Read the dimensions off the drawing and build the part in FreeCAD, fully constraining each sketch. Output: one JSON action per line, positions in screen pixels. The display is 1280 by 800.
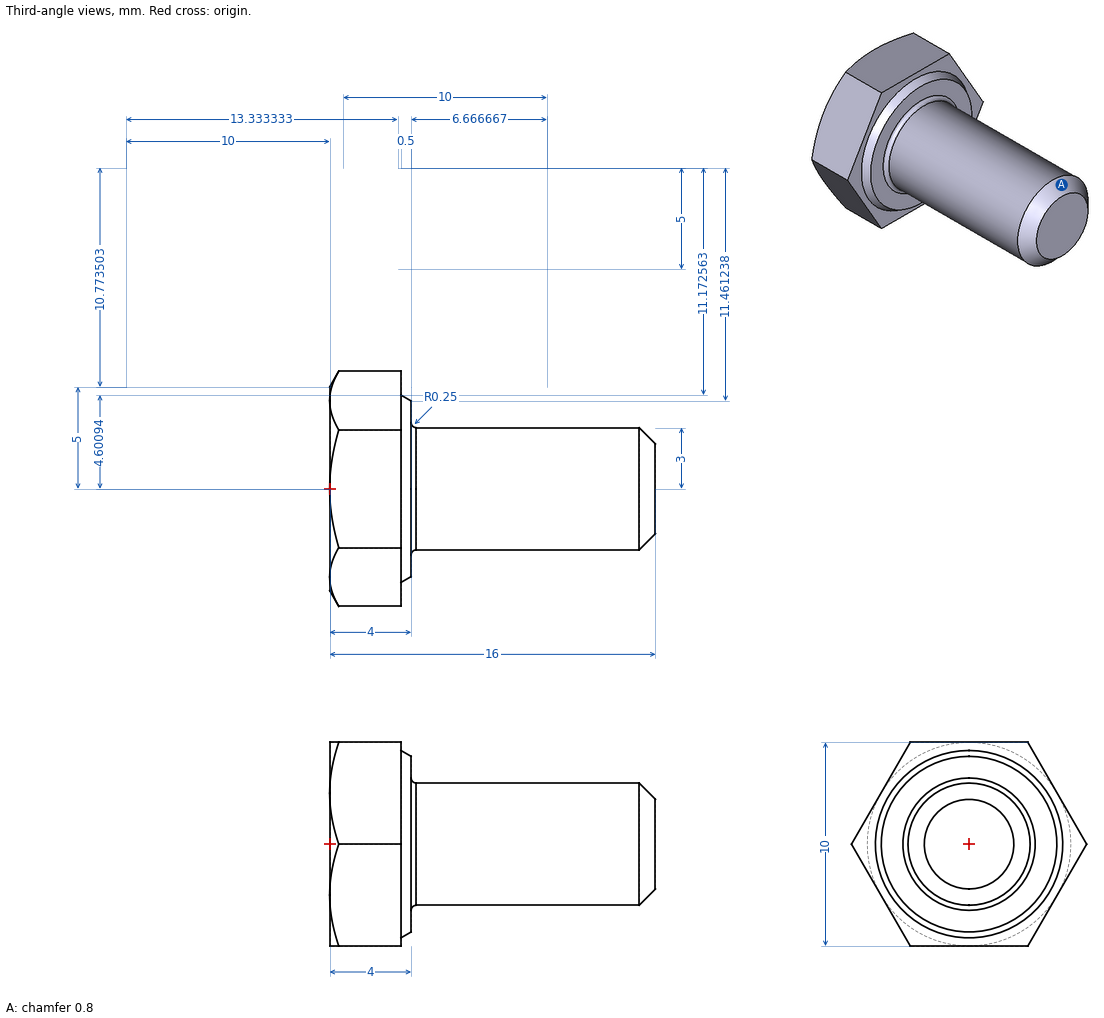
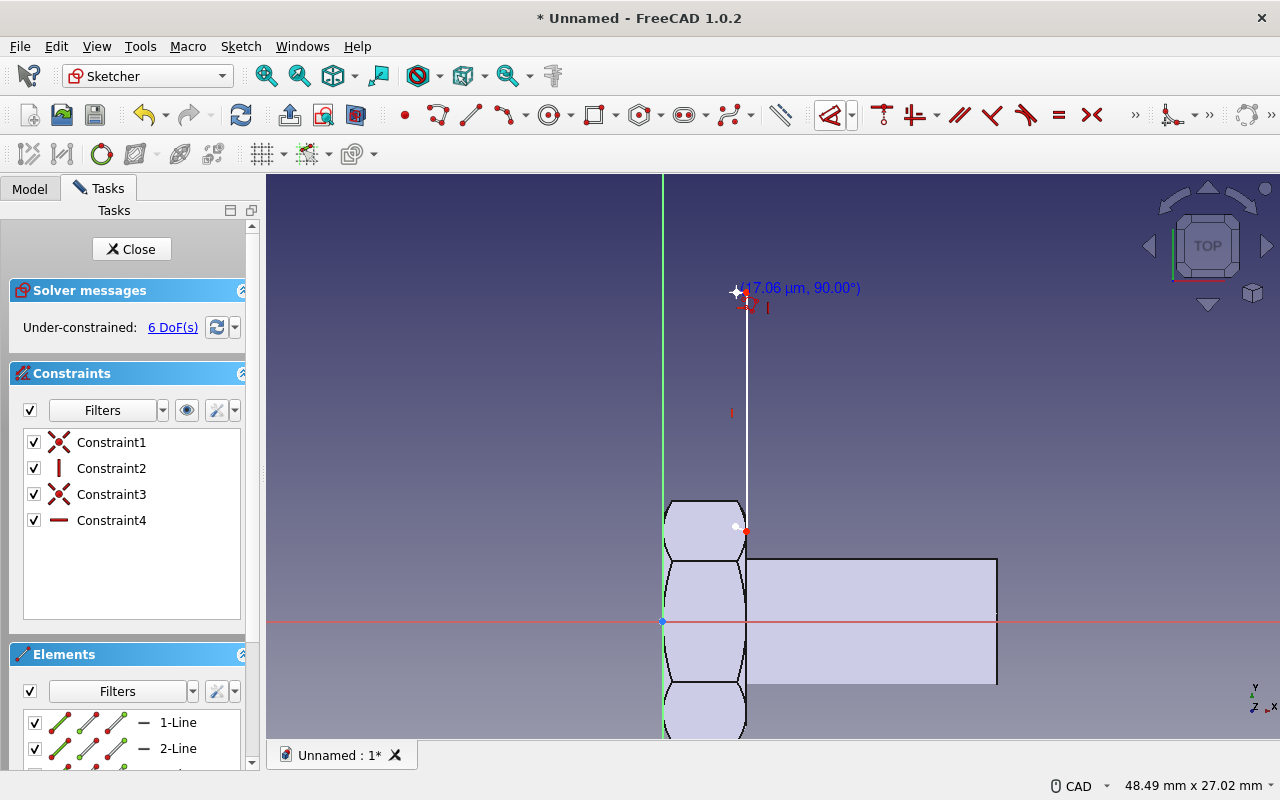
{"action": "scroll", "coordinate": [736, 525], "scroll_direction": "up", "scroll_amount": 5}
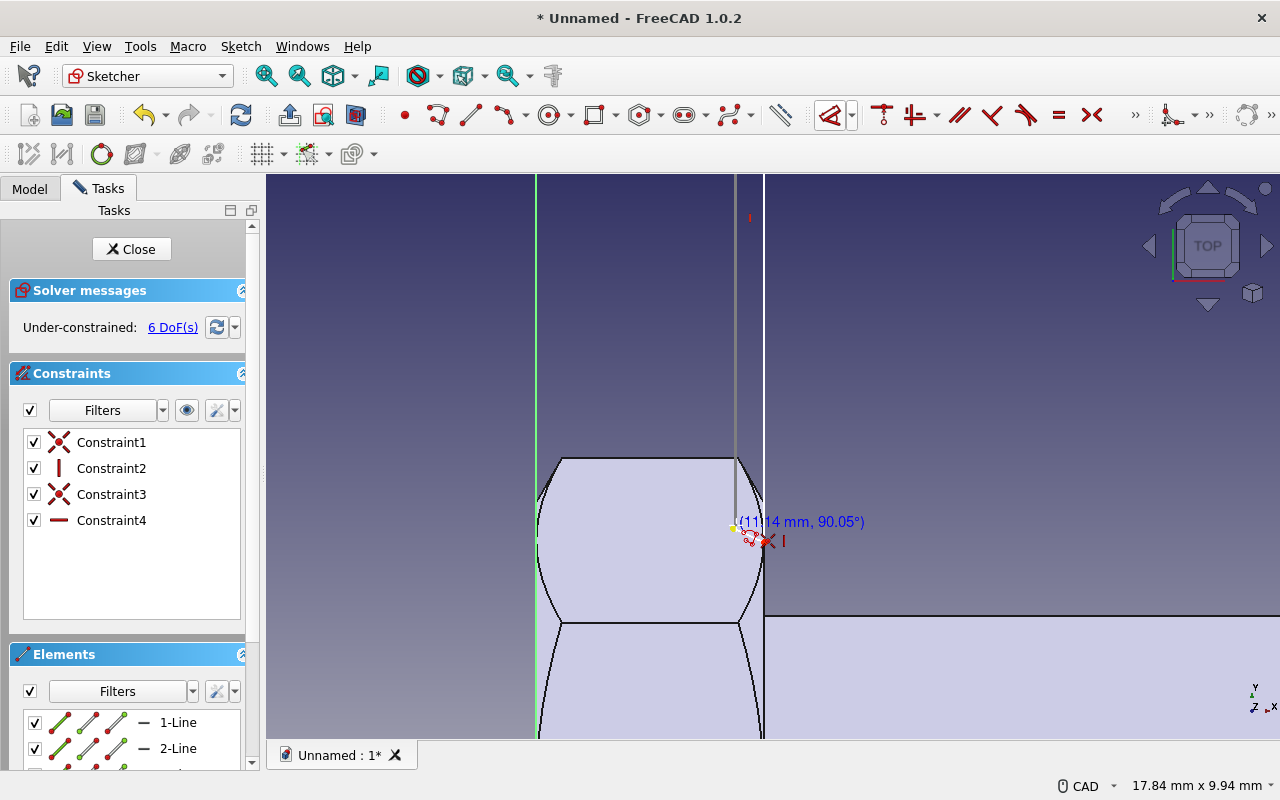
{"action": "left_click", "coordinate": [734, 529]}
{"action": "key", "text": "Escape"}
{"action": "key", "text": "Escape"}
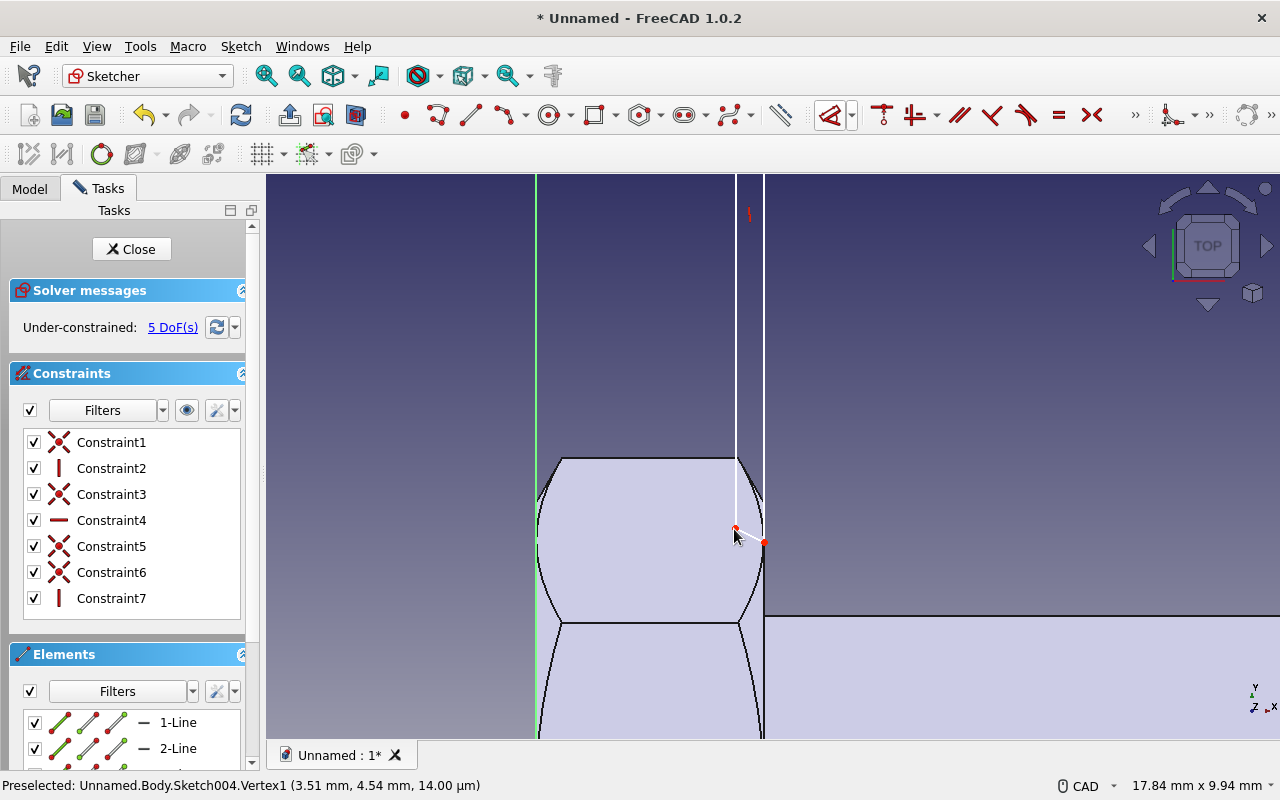
{"action": "left_click", "coordinate": [764, 543]}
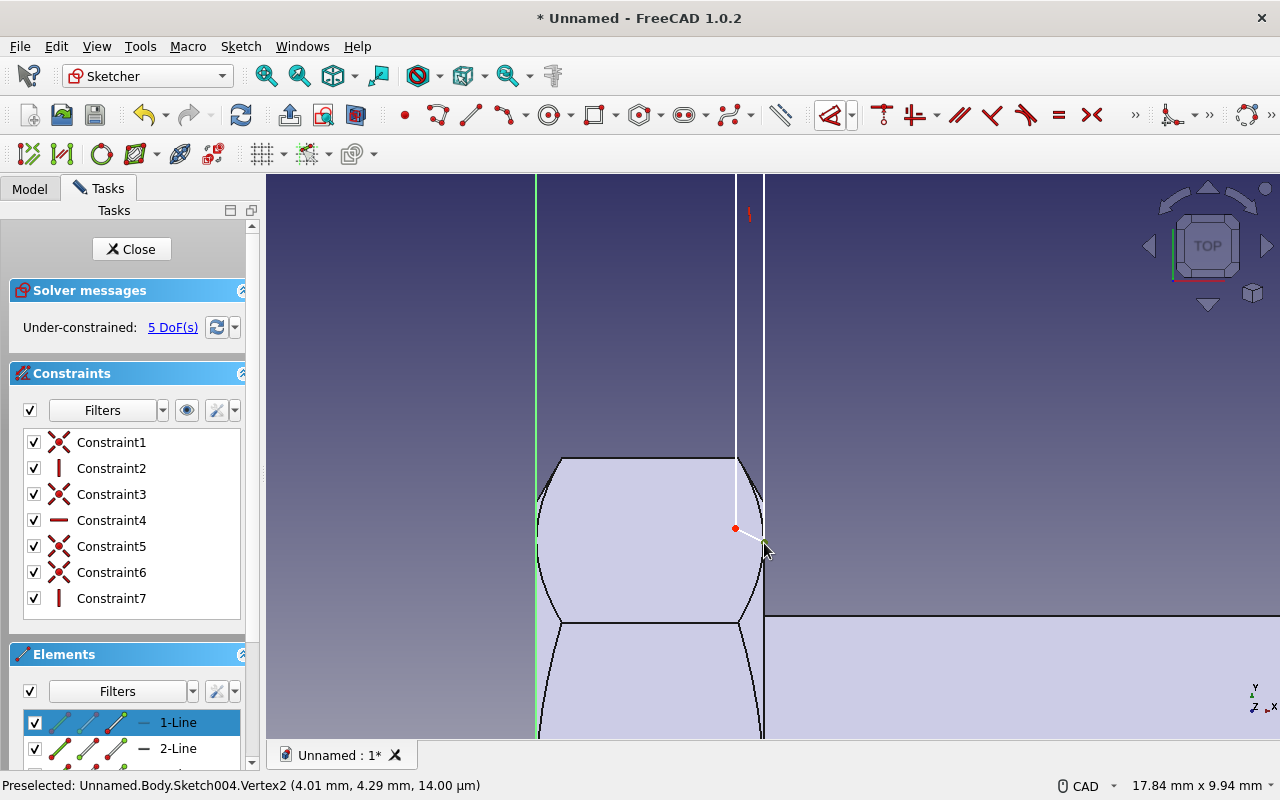
{"action": "left_click", "coordinate": [852, 116]}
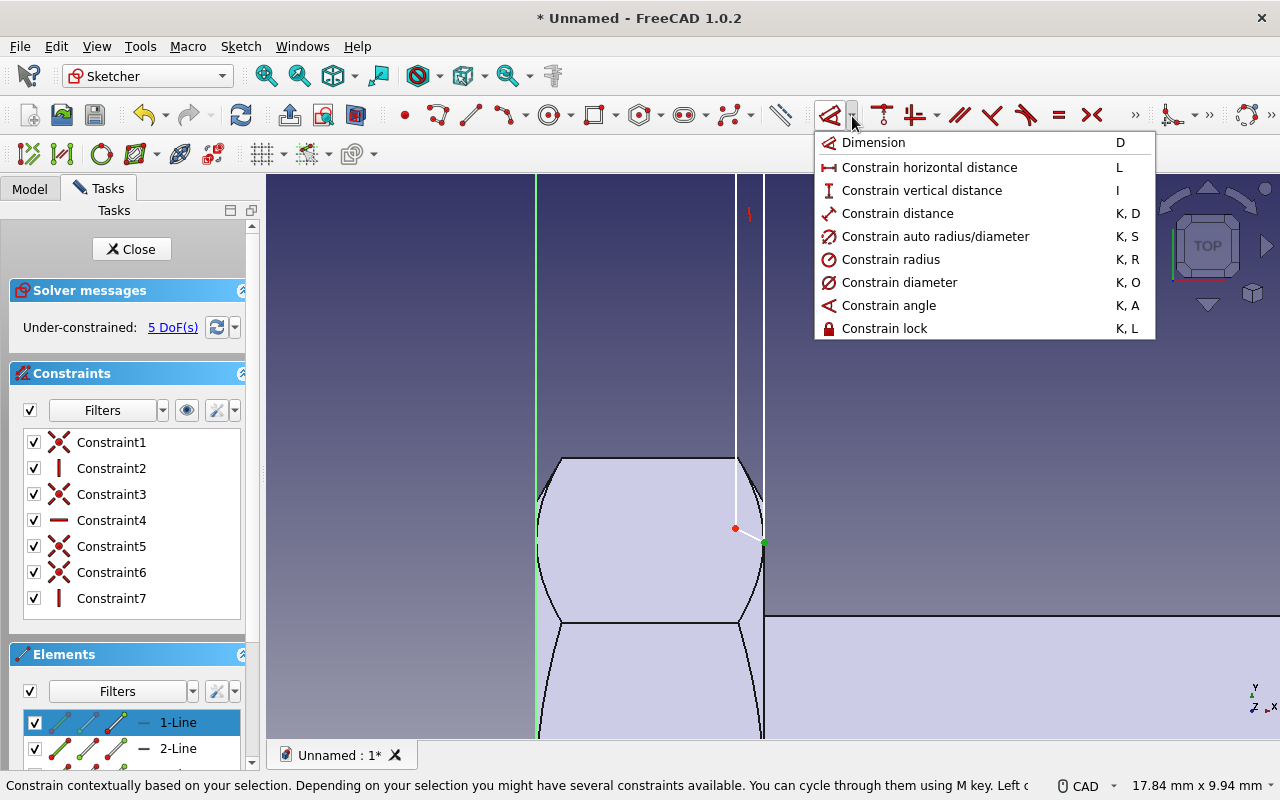
{"action": "left_click", "coordinate": [985, 168]}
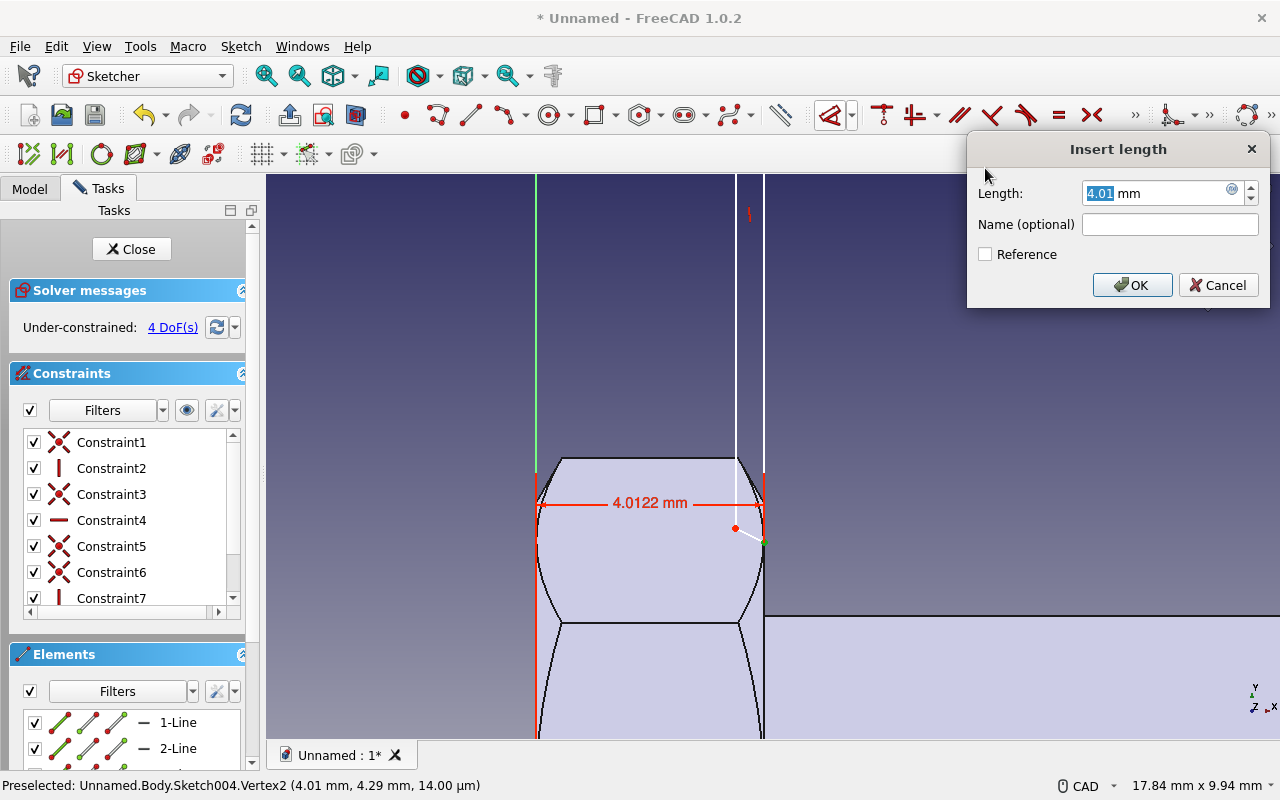
{"action": "type", "text": "4"}
{"action": "key", "text": "Return"}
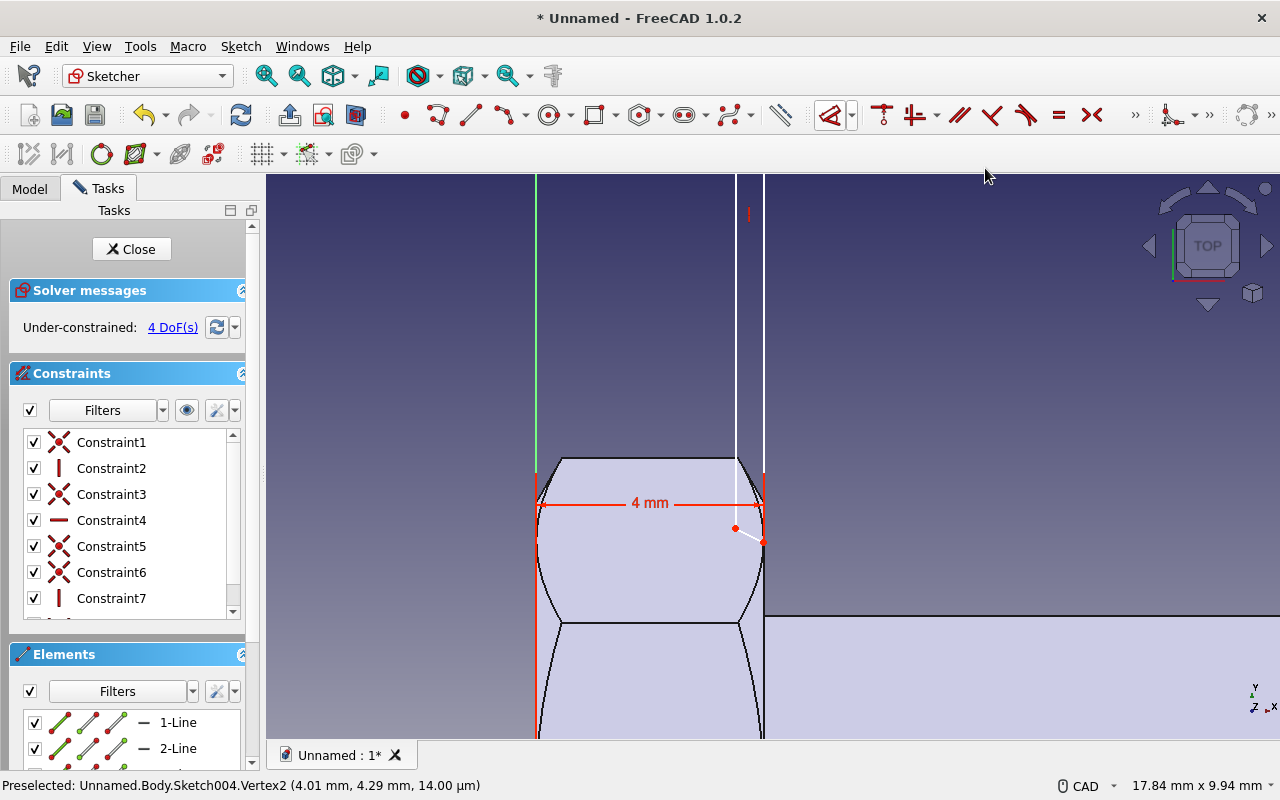
{"action": "scroll", "coordinate": [736, 525], "scroll_direction": "down", "scroll_amount": 5}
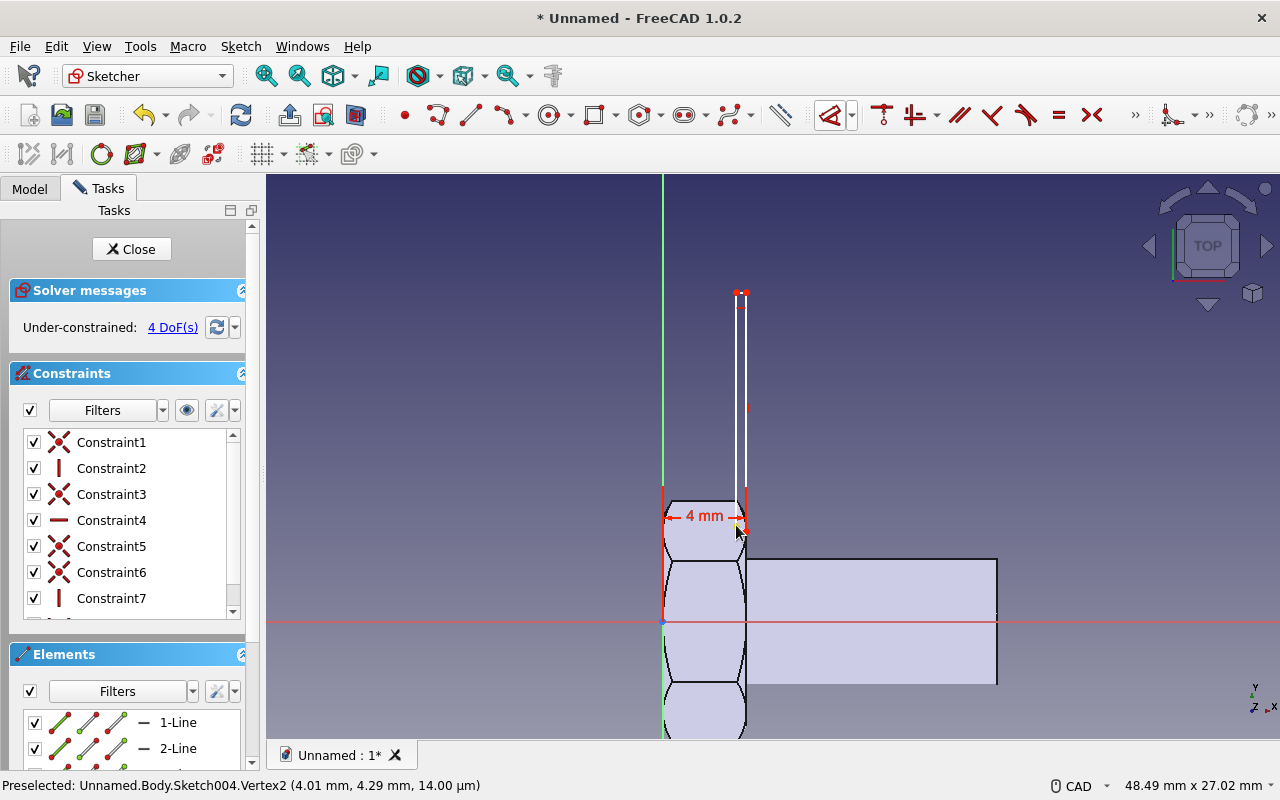
{"action": "scroll", "coordinate": [742, 293], "scroll_direction": "up", "scroll_amount": 7}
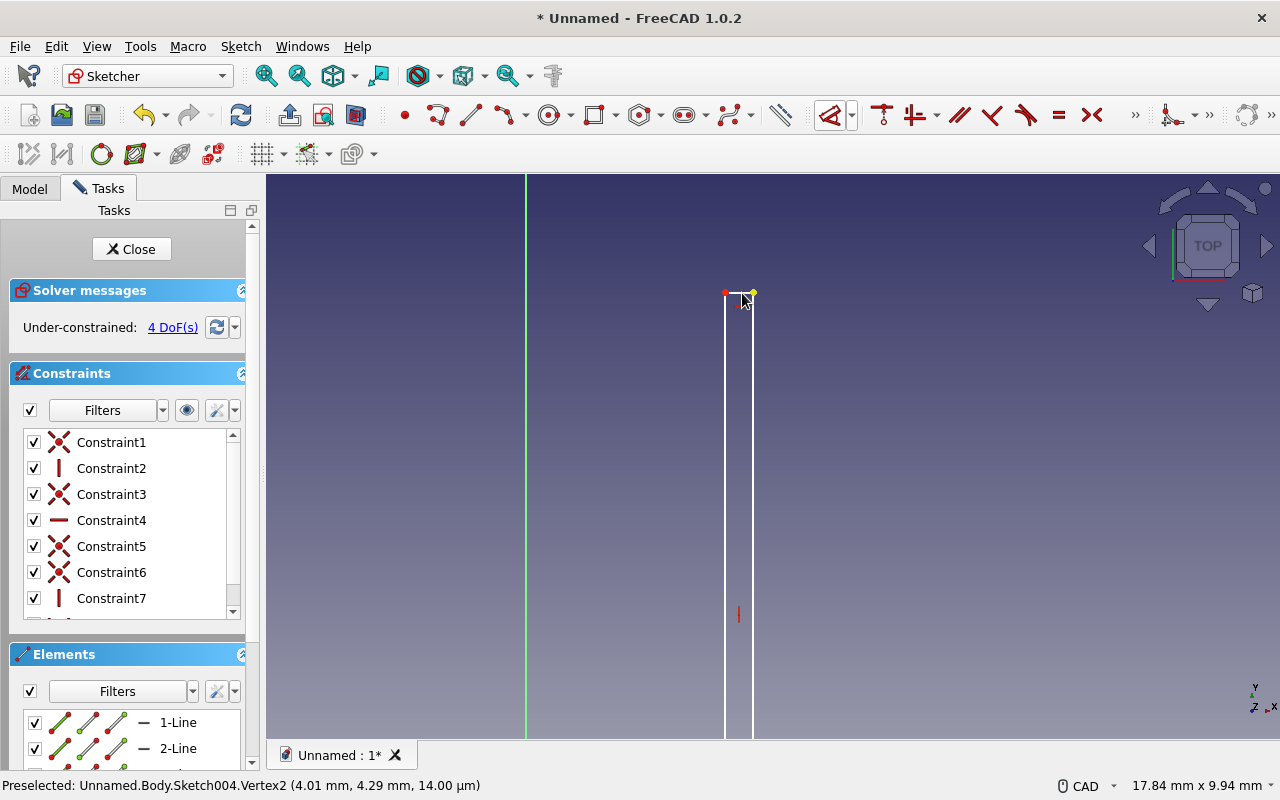
{"action": "left_click", "coordinate": [742, 292]}